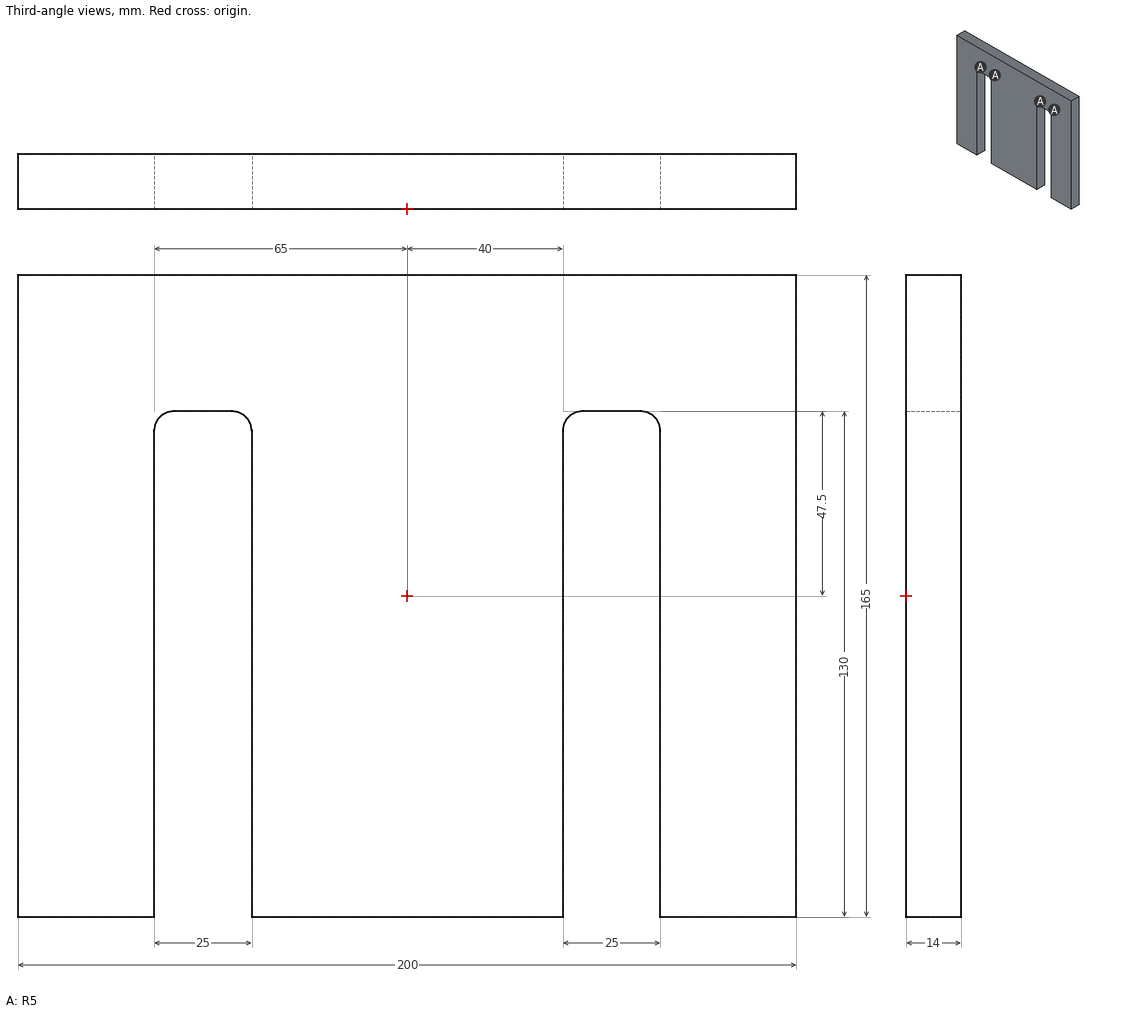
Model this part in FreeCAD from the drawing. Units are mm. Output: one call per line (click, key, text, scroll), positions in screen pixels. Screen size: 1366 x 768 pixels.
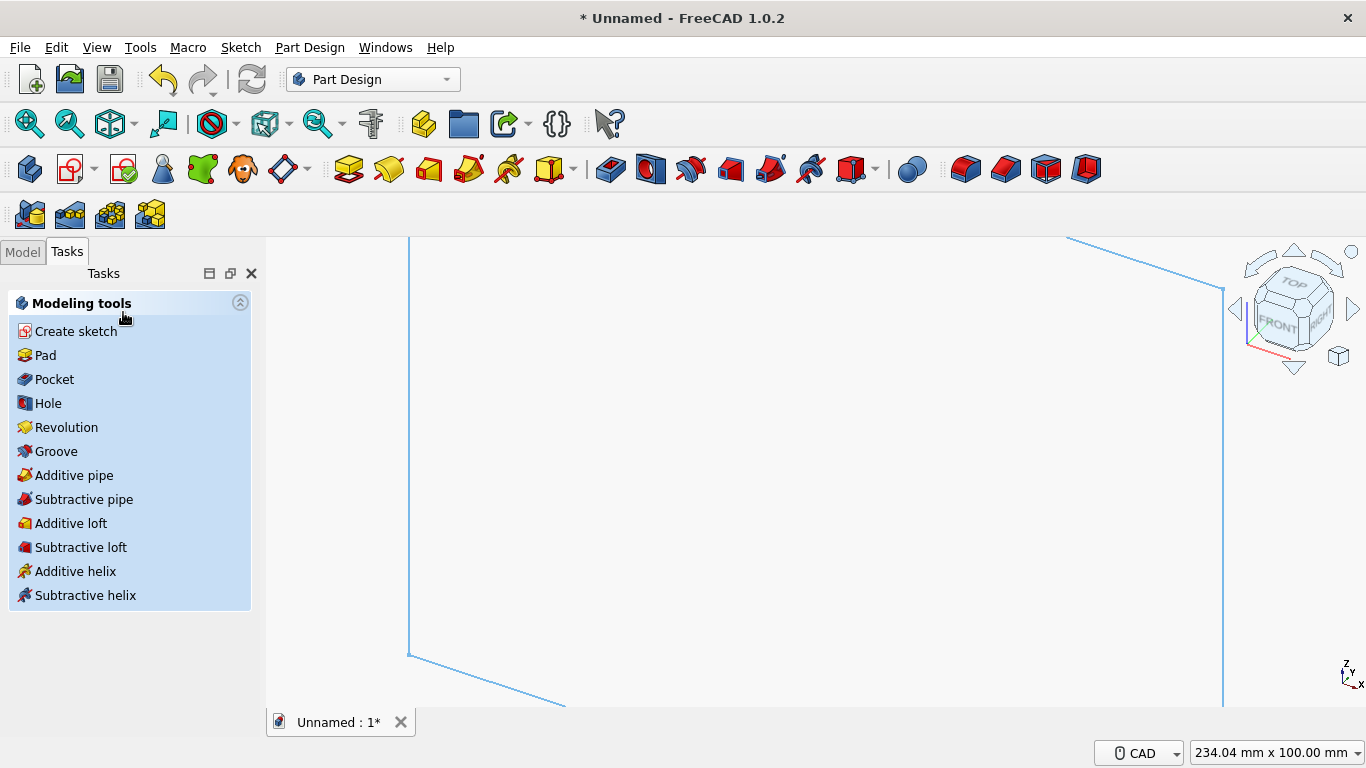
click(350, 170)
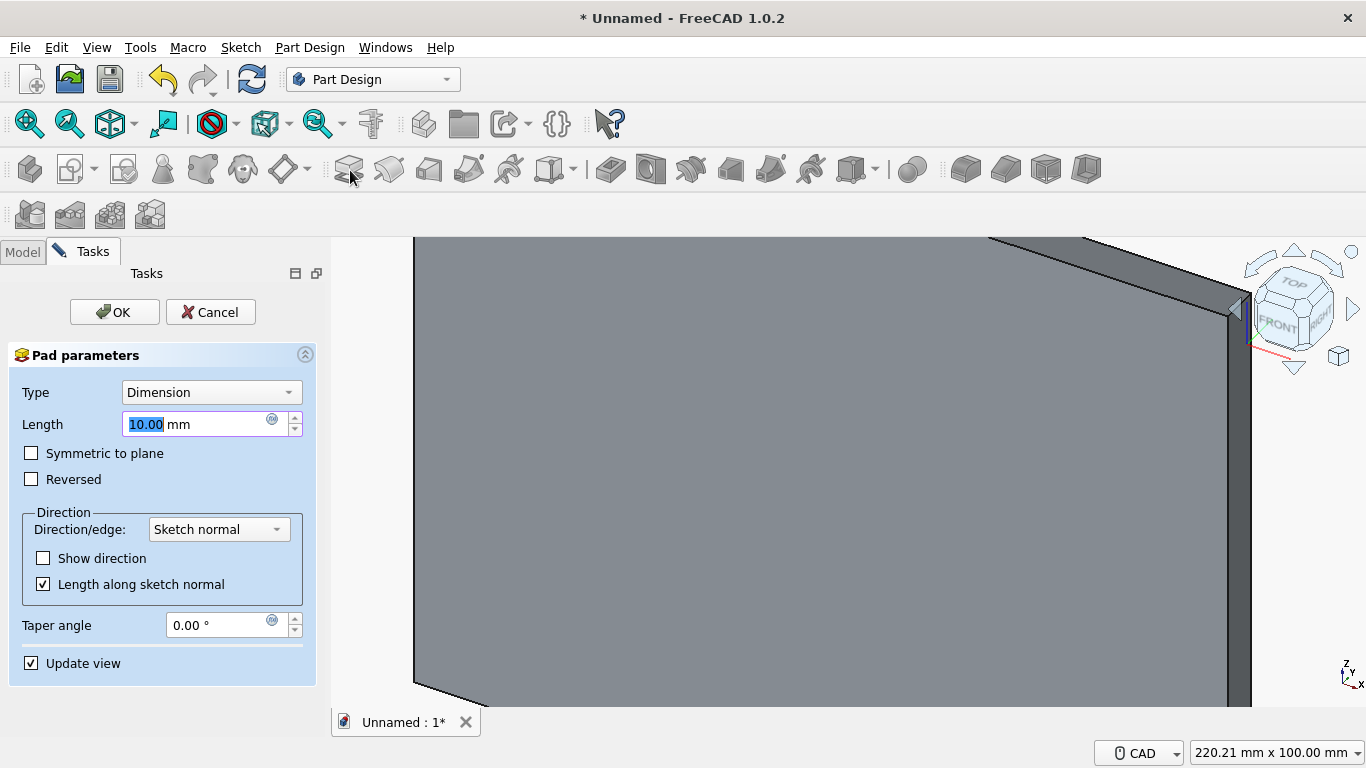
text(14)
key(Tab)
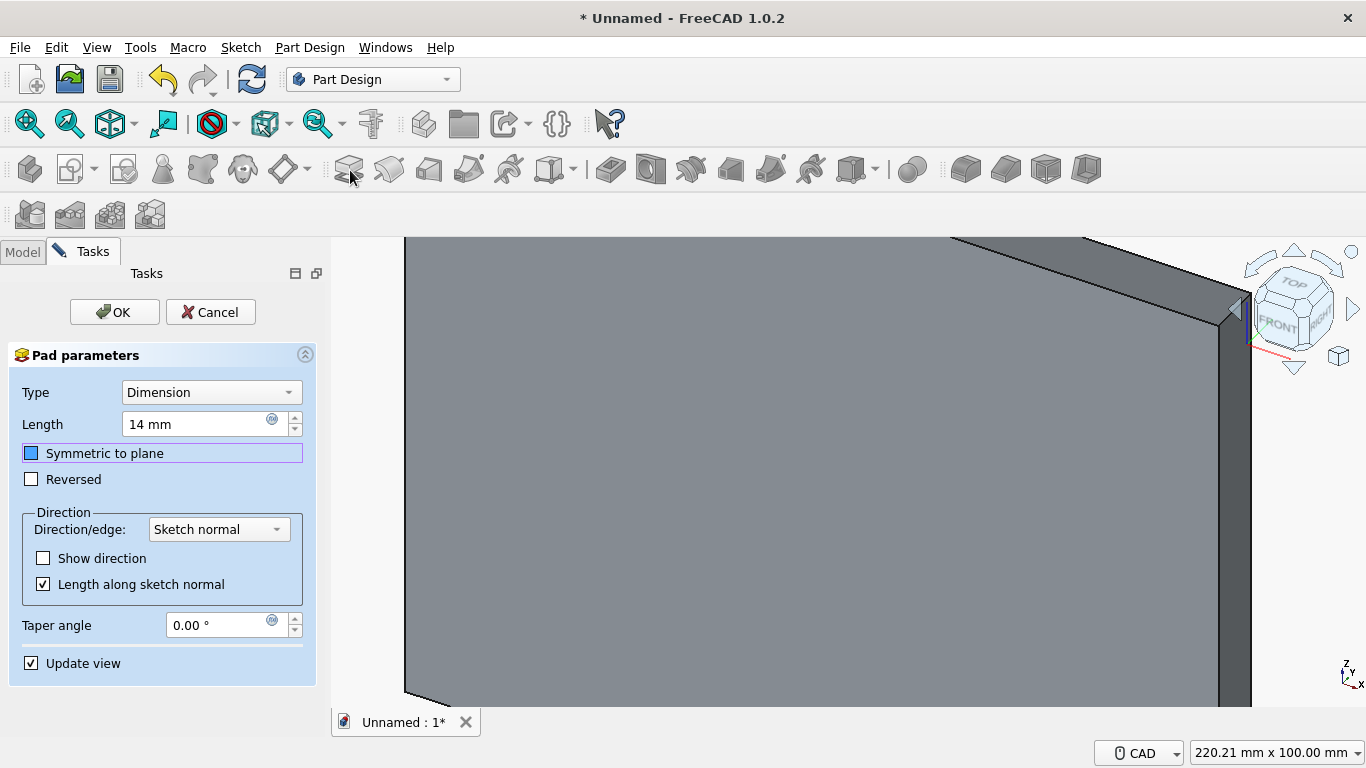
click(30, 479)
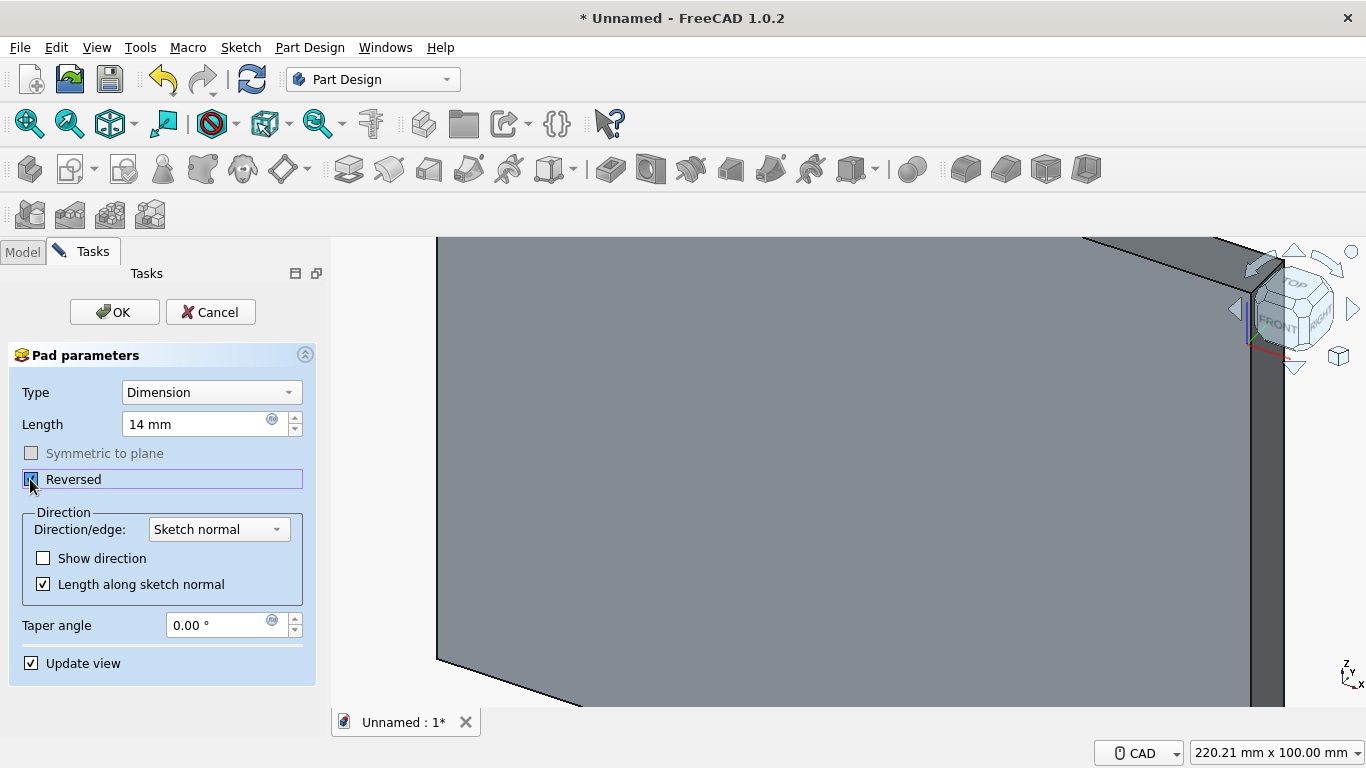
click(115, 312)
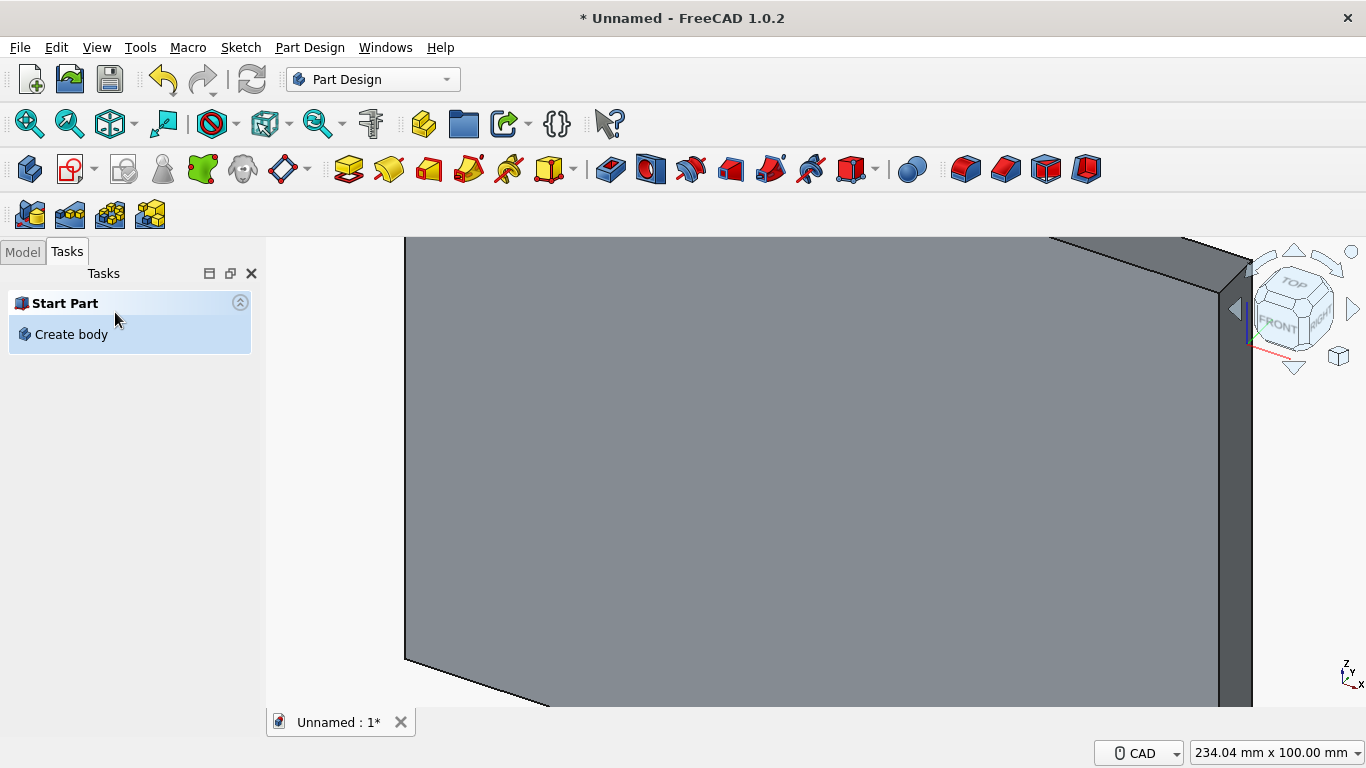
click(30, 124)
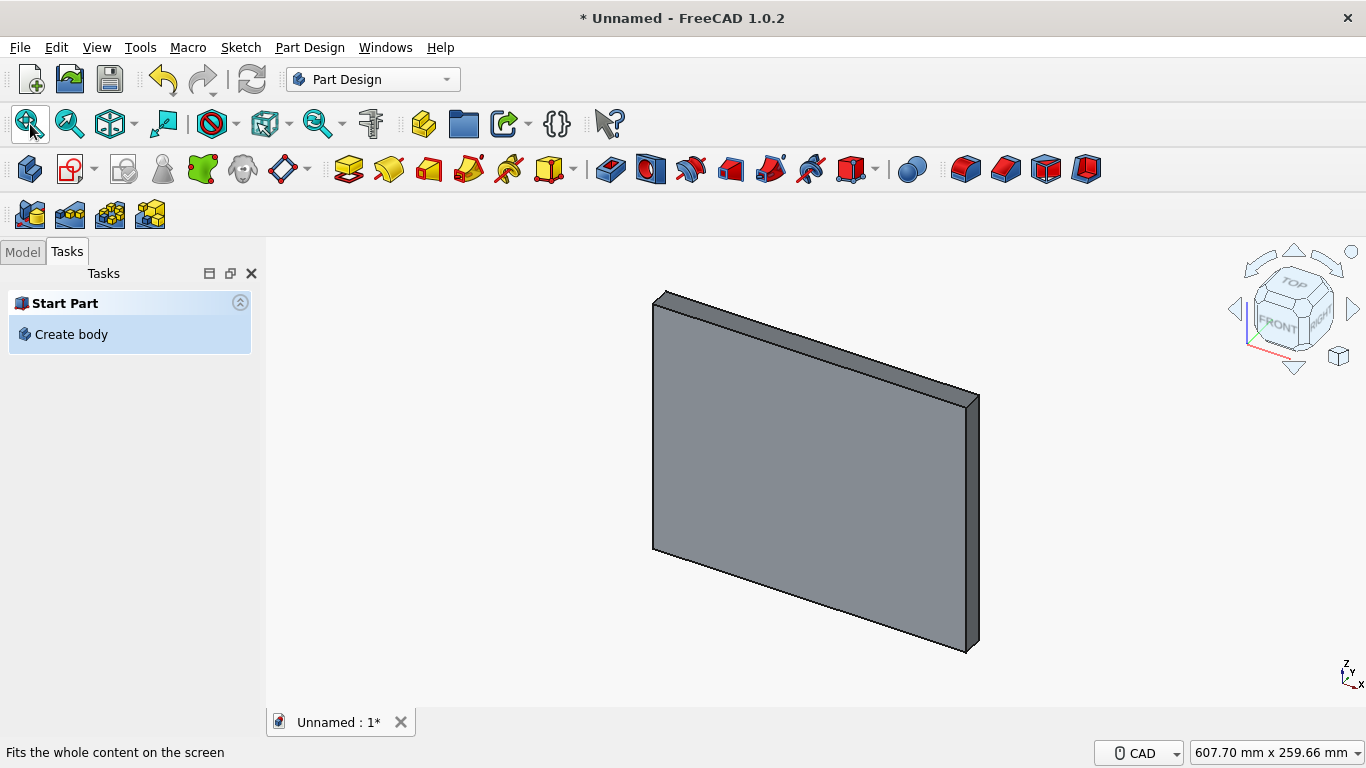
click(70, 170)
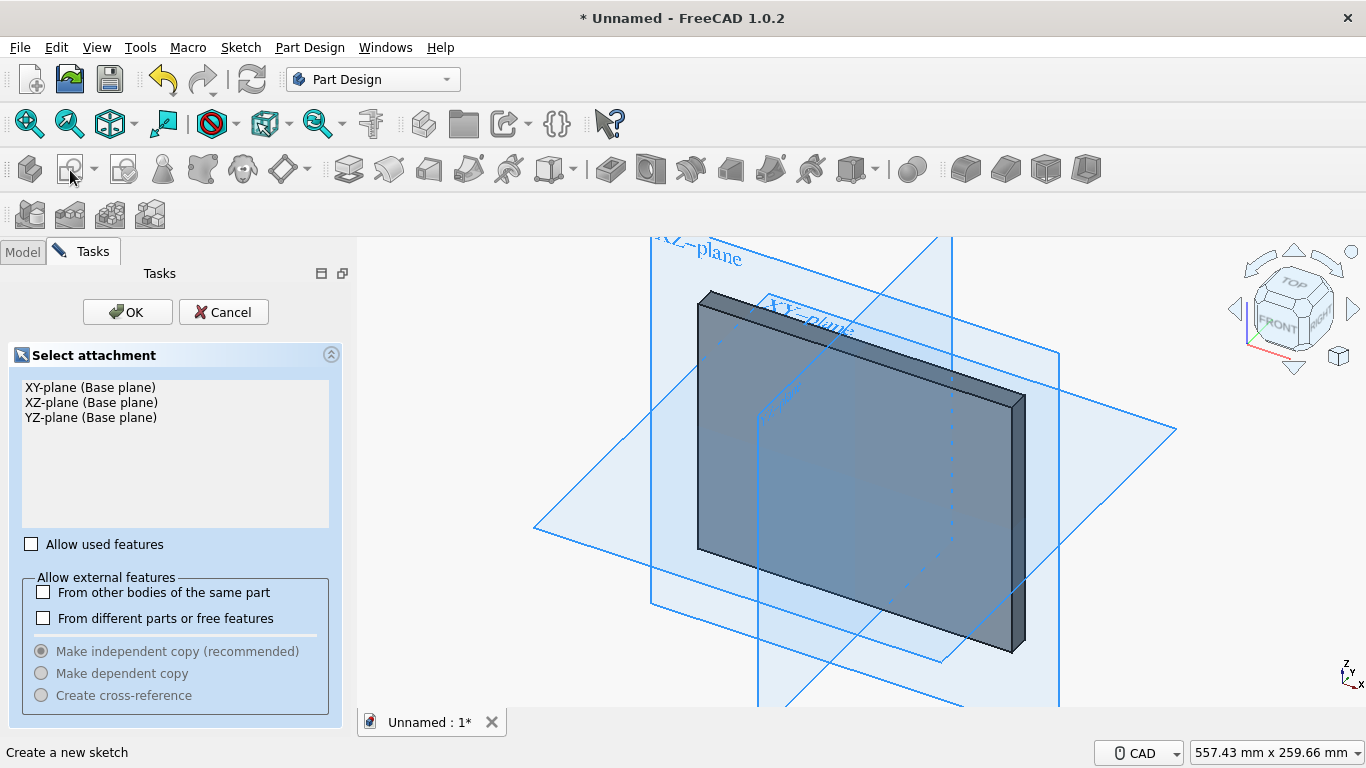
click(82, 402)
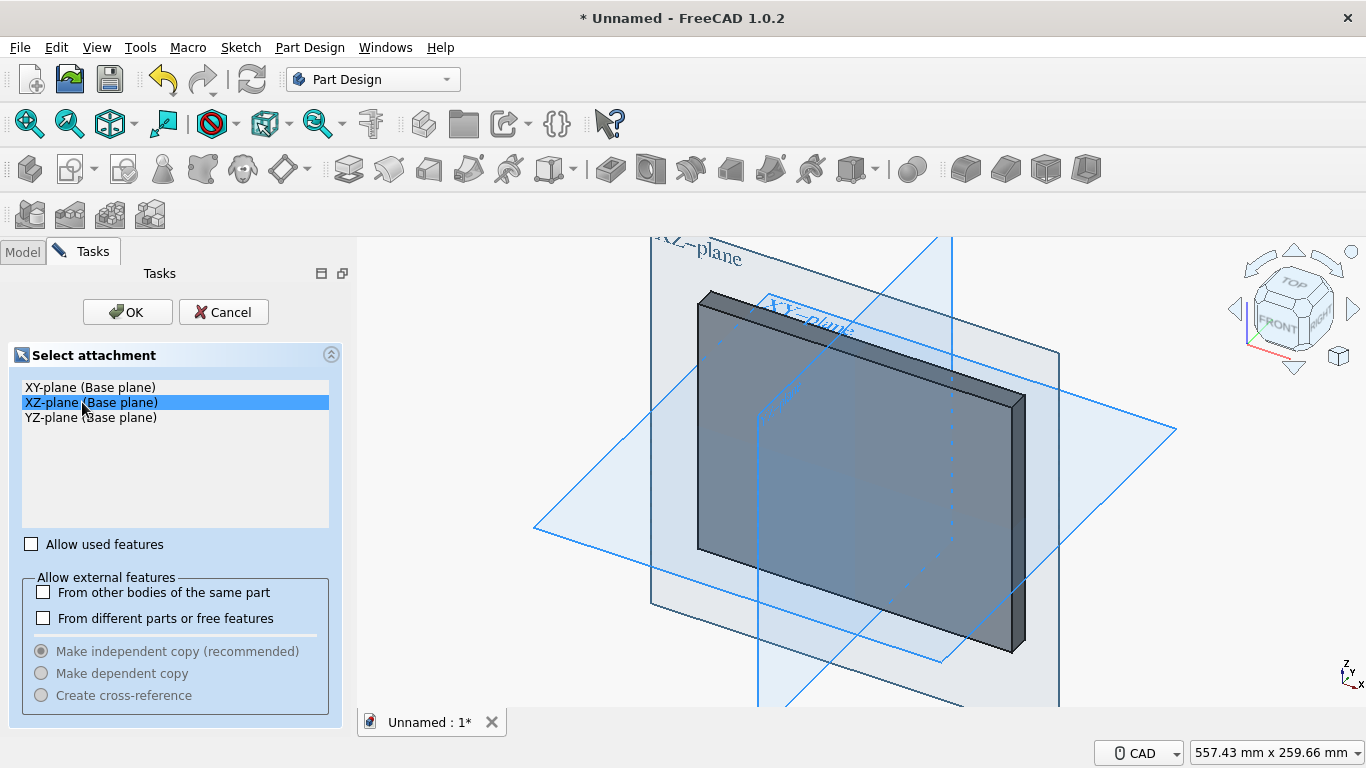
click(128, 312)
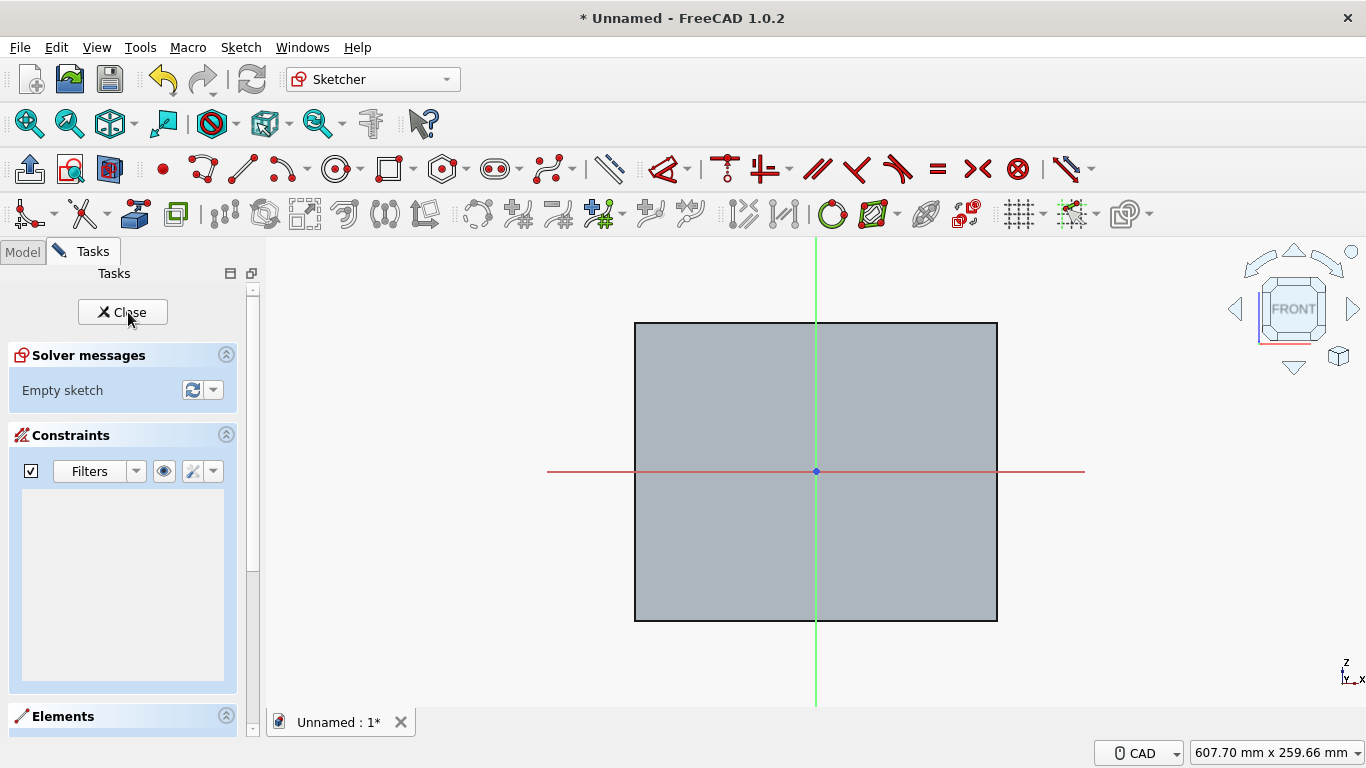
click(390, 170)